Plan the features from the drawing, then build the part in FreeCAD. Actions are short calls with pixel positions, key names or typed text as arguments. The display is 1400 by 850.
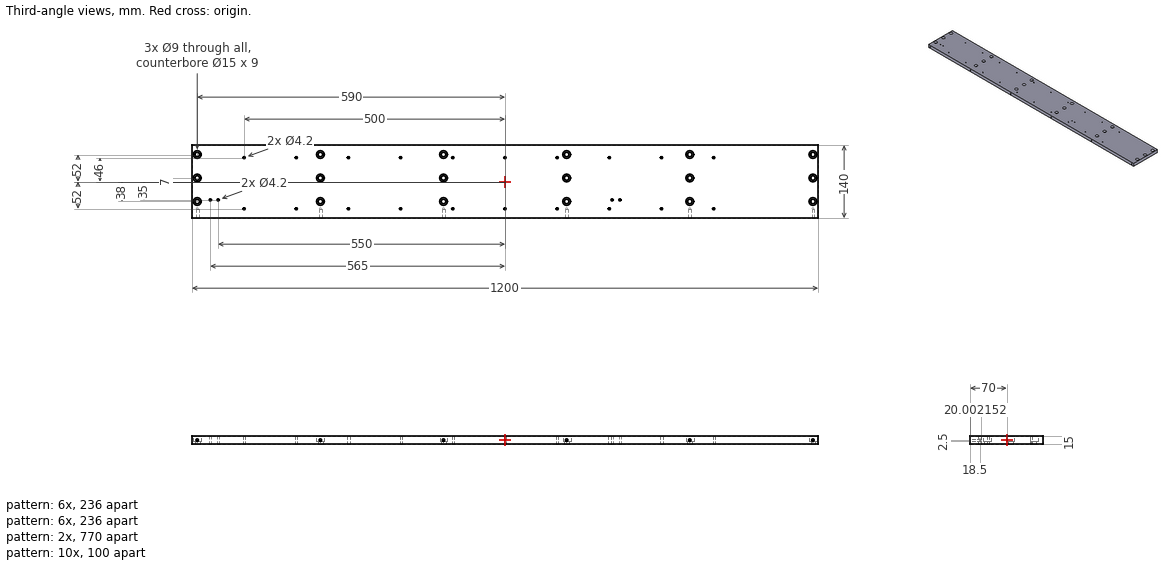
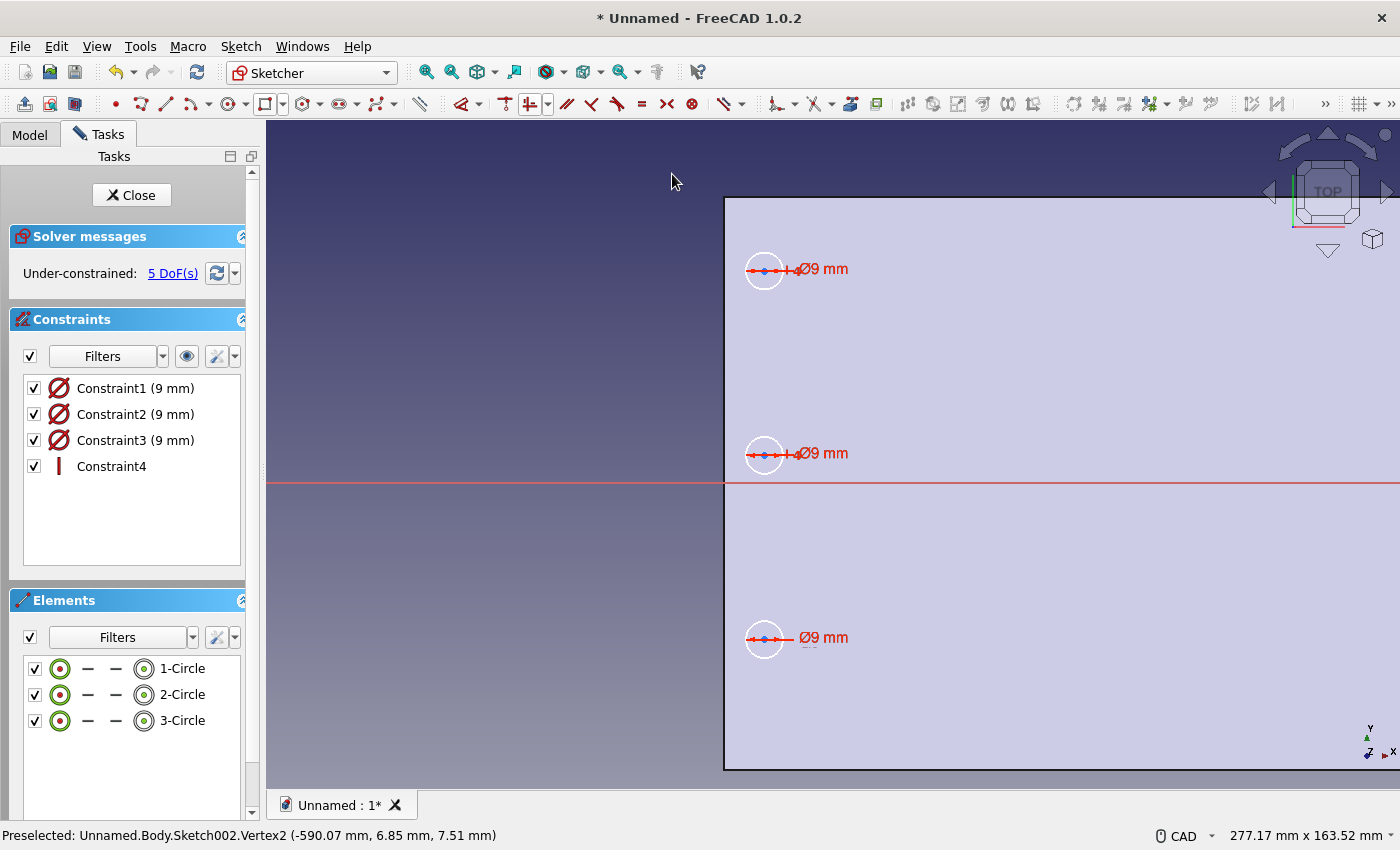
click(764, 455)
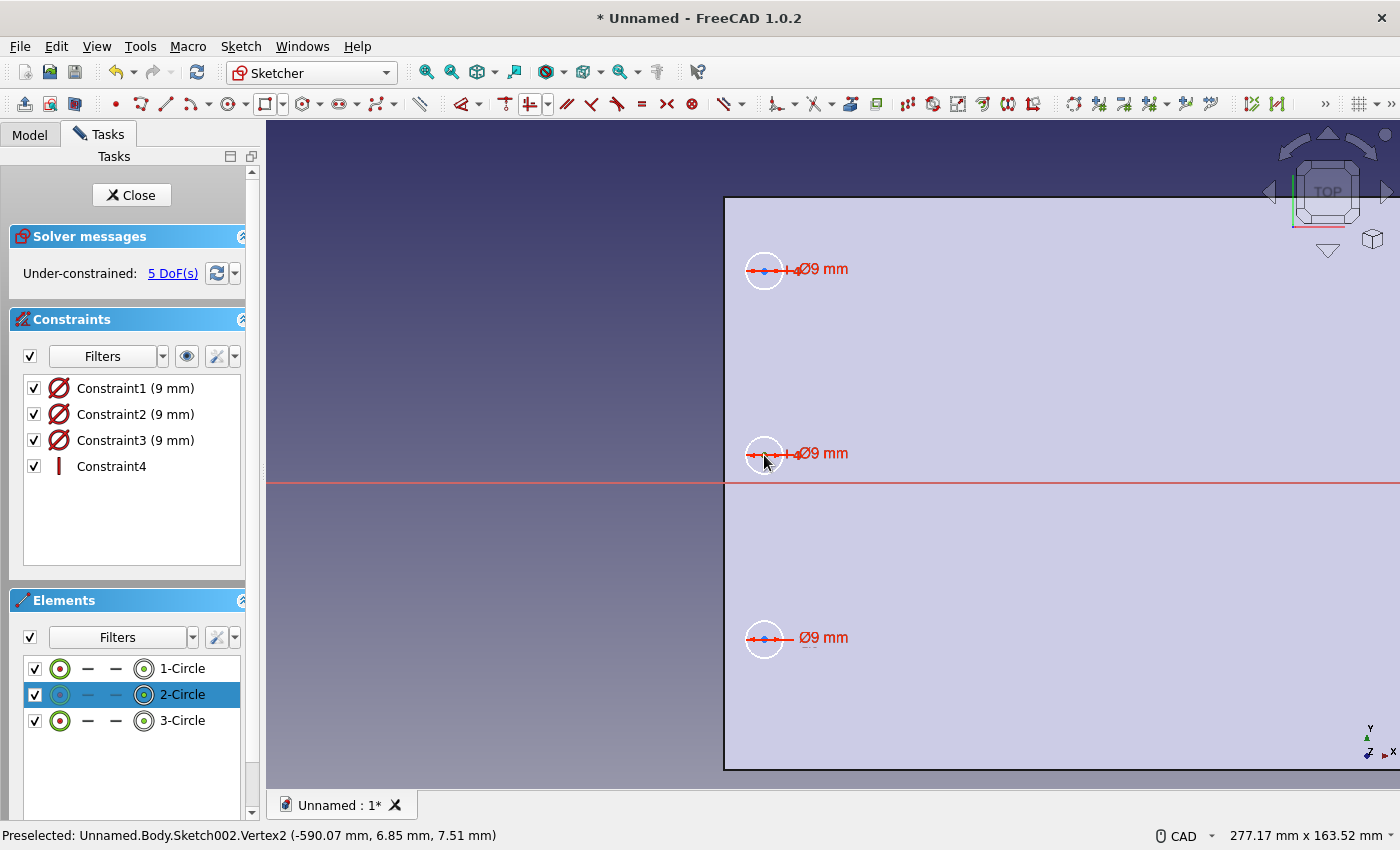
click(764, 640)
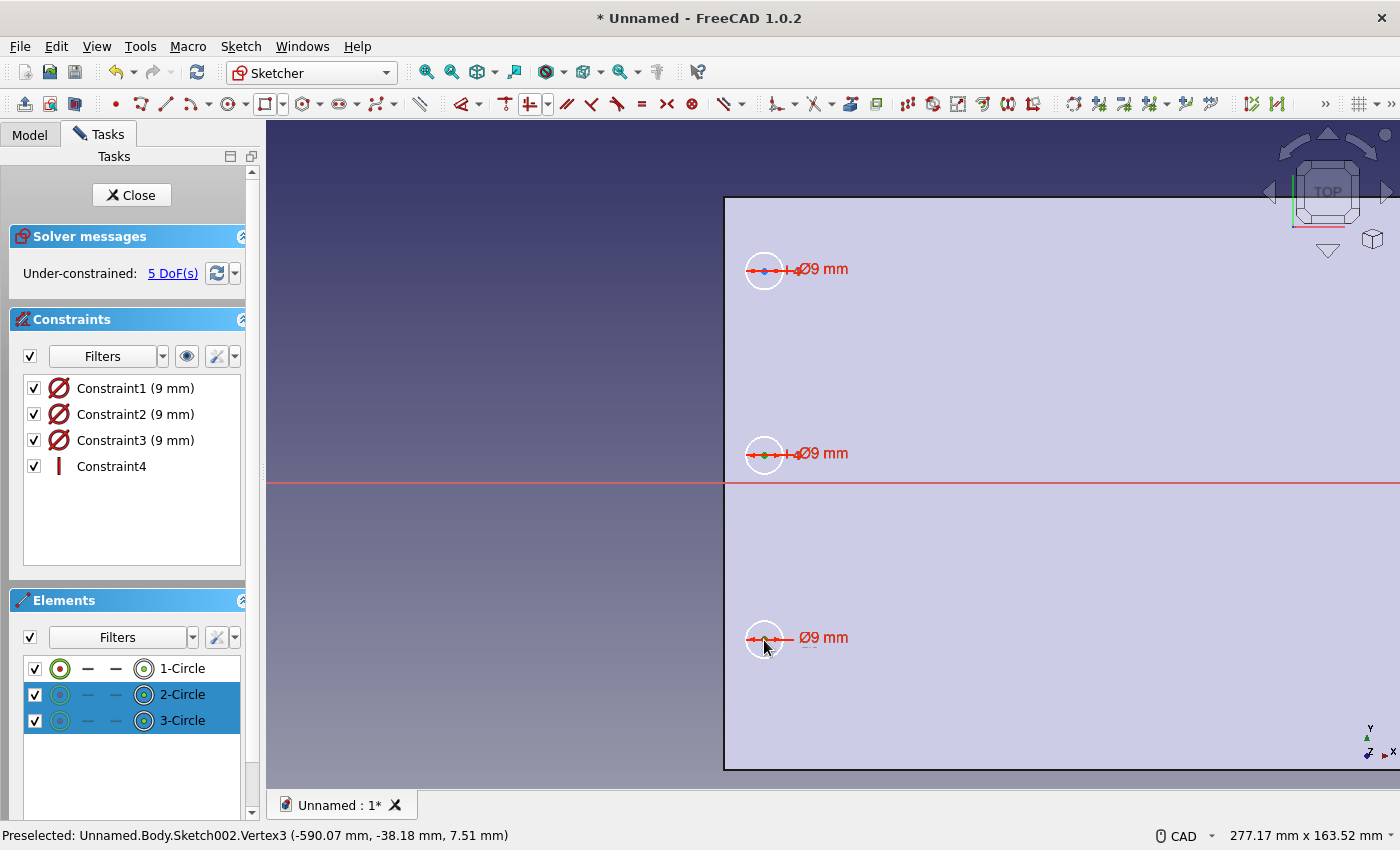
key(v)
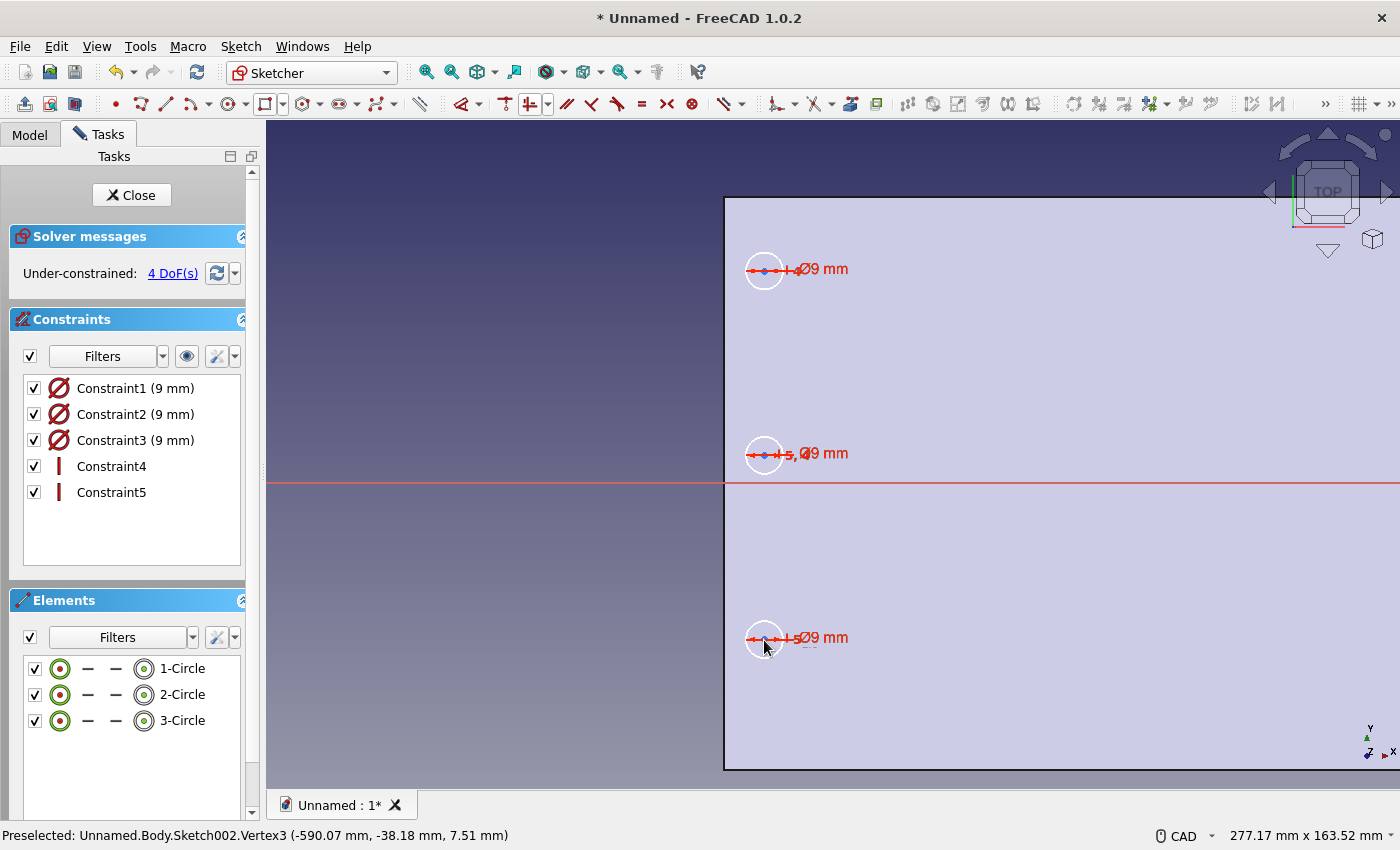
key(d)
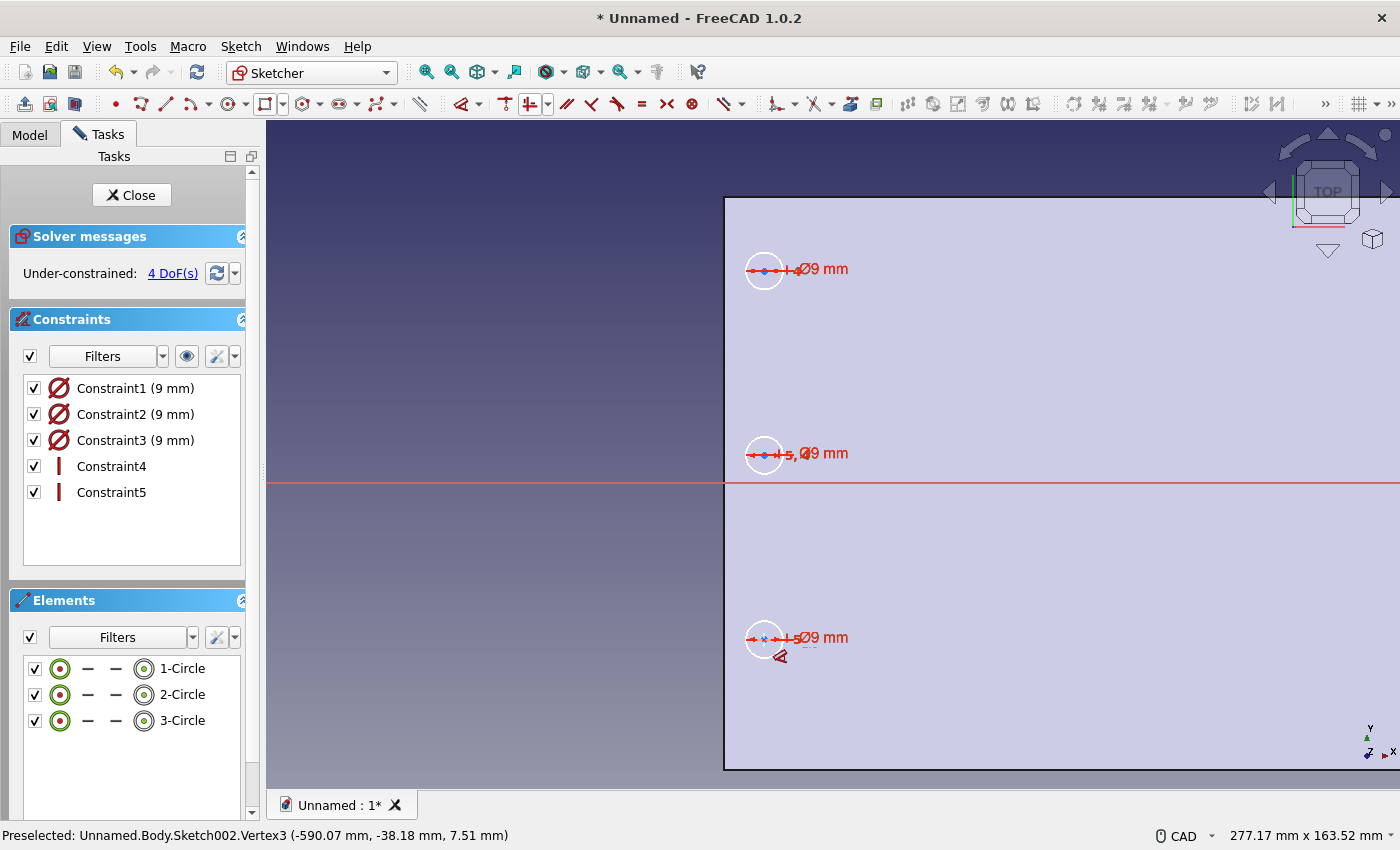
scroll(764, 455, up, 2)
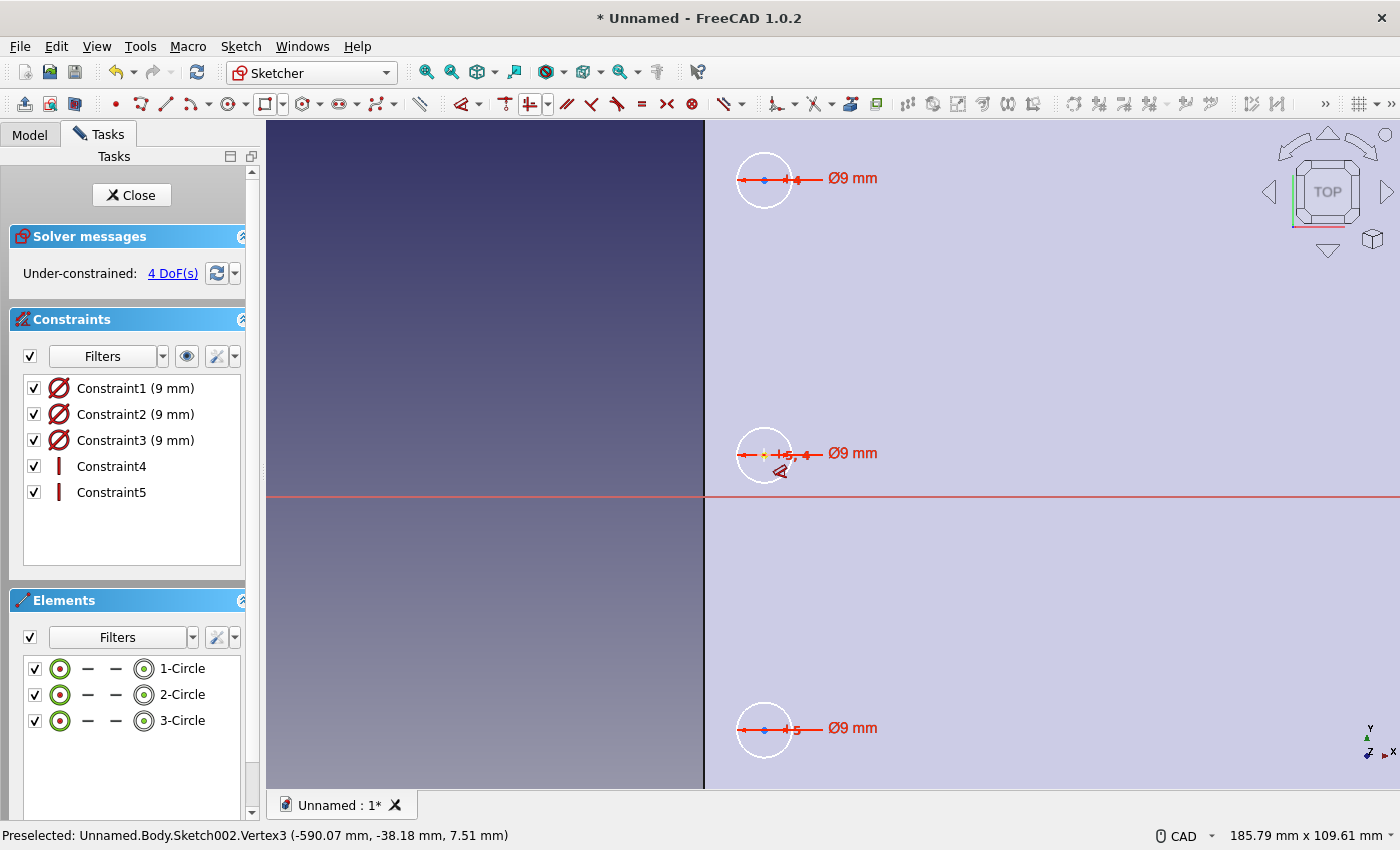
click(764, 455)
click(706, 476)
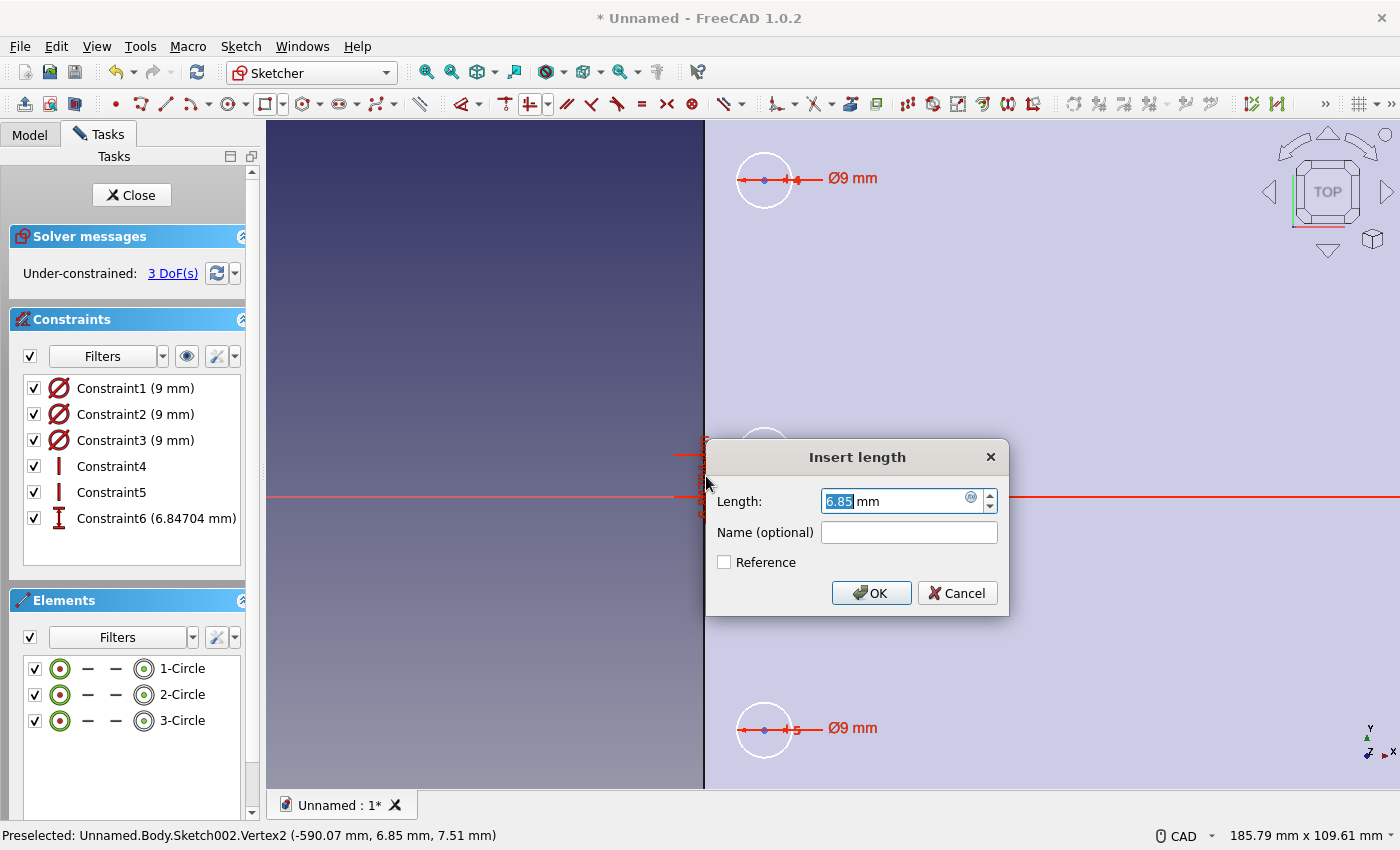
text(7)
key(Return)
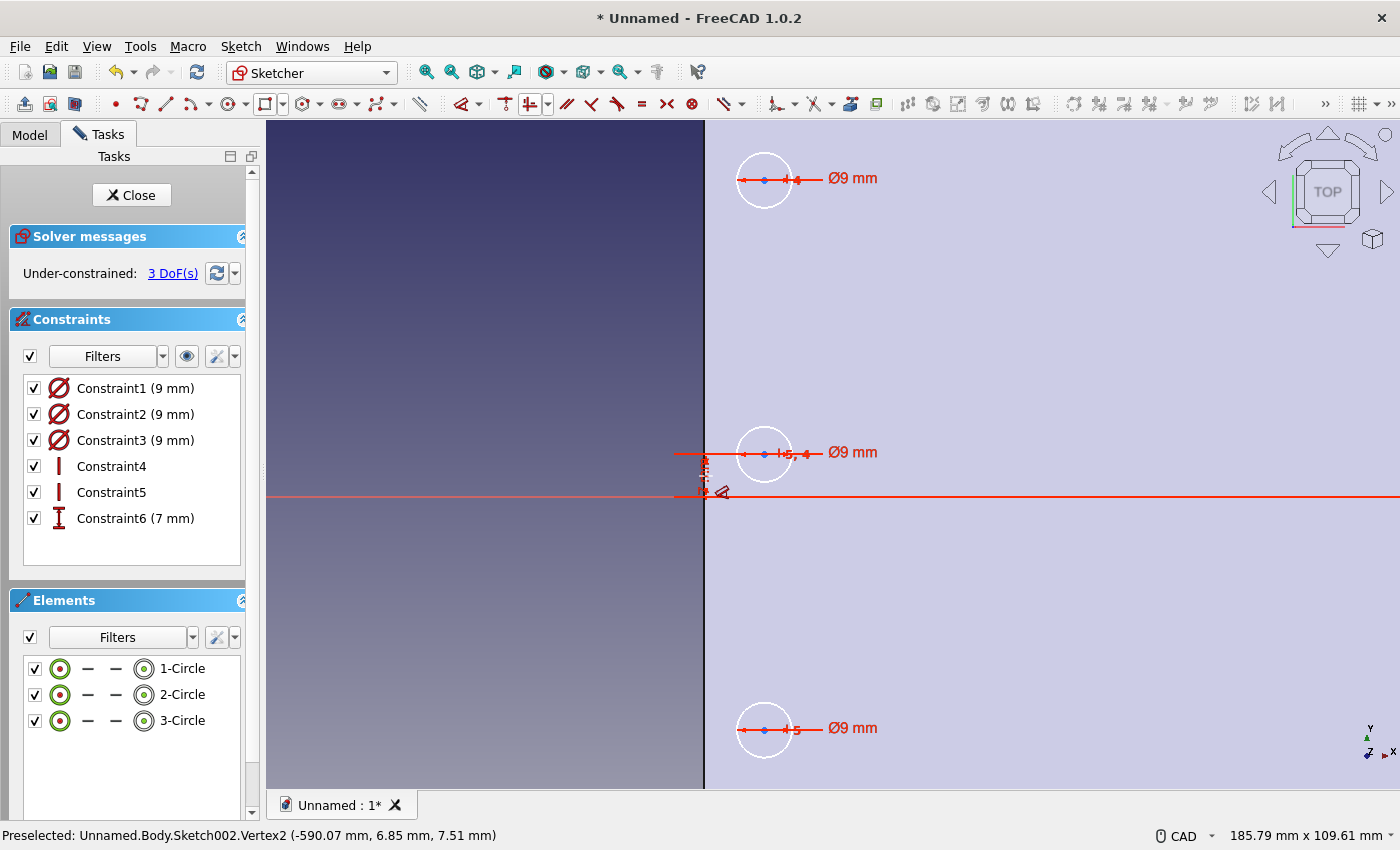
click(764, 180)
click(730, 339)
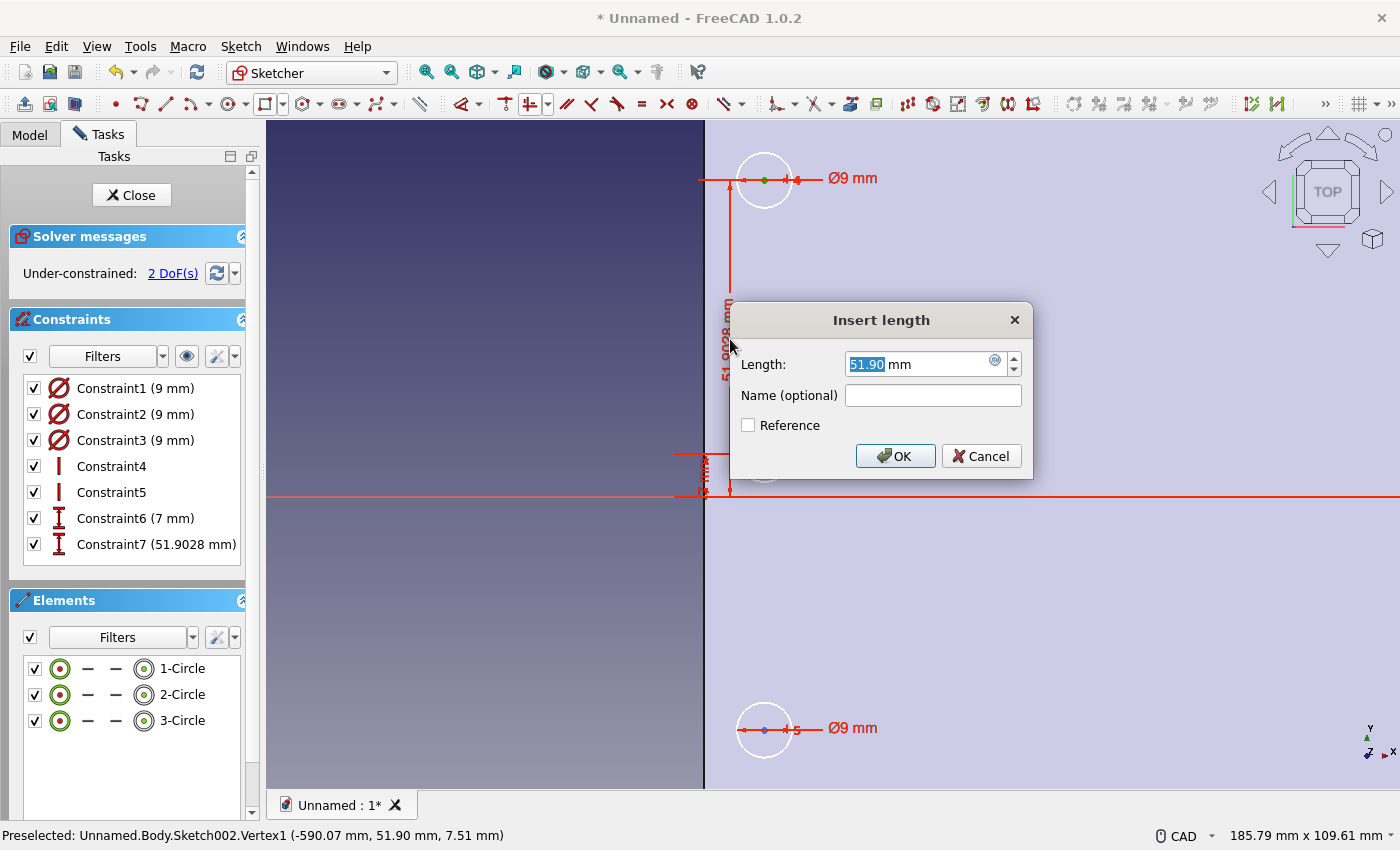
text(52)
key(Return)